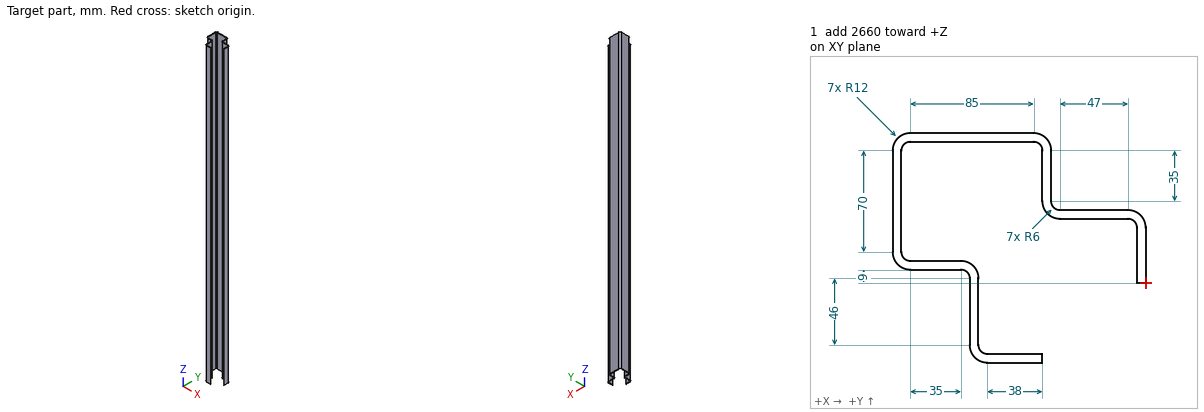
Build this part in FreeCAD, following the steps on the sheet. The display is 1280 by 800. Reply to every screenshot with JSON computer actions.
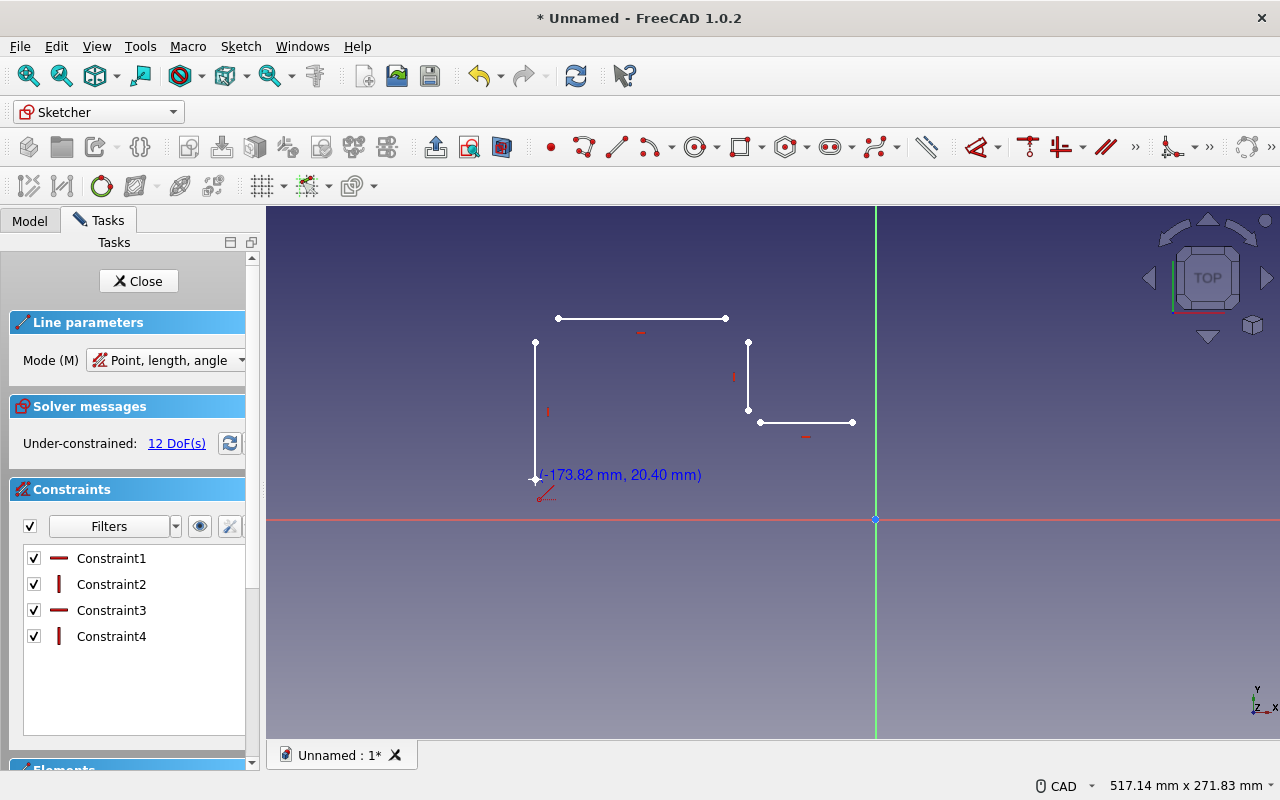
{"action": "left_click", "coordinate": [558, 502]}
{"action": "left_click", "coordinate": [627, 502]}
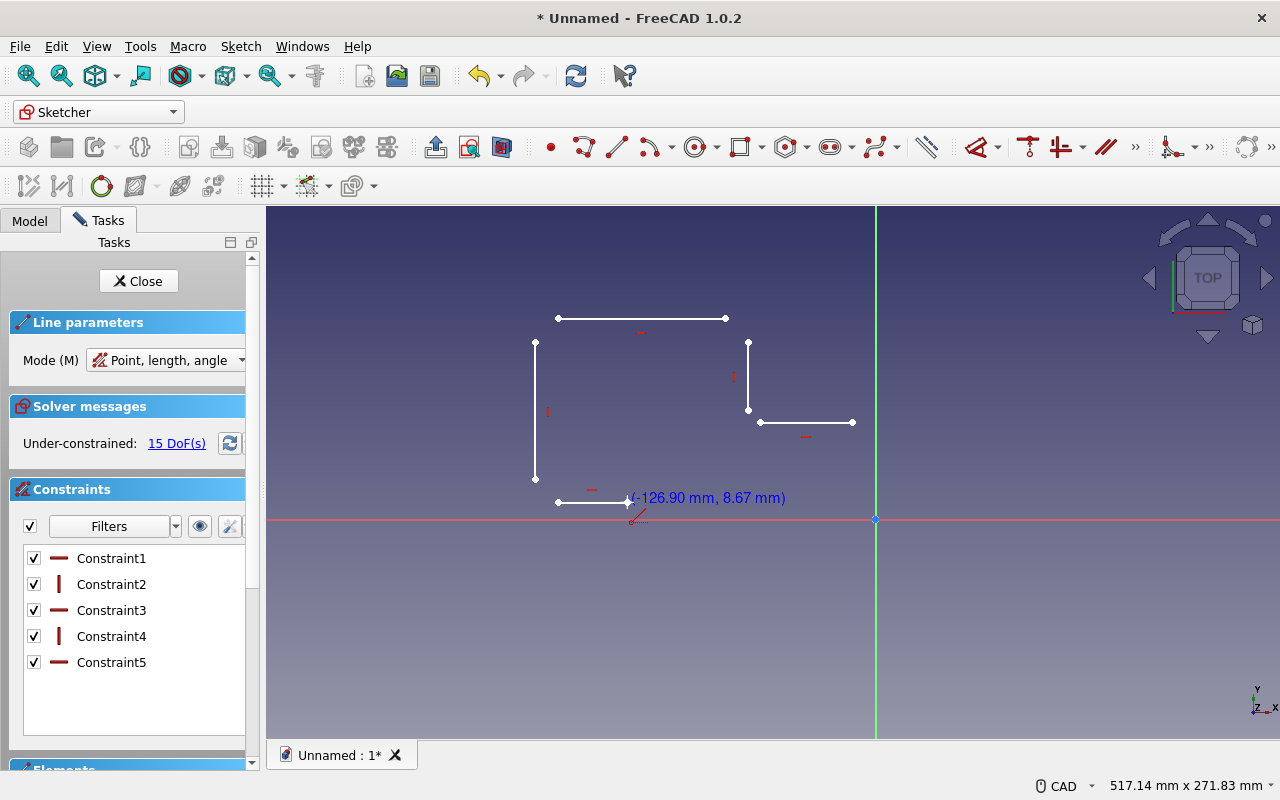
{"action": "scroll", "coordinate": [639, 514], "scroll_direction": "up", "scroll_amount": 5}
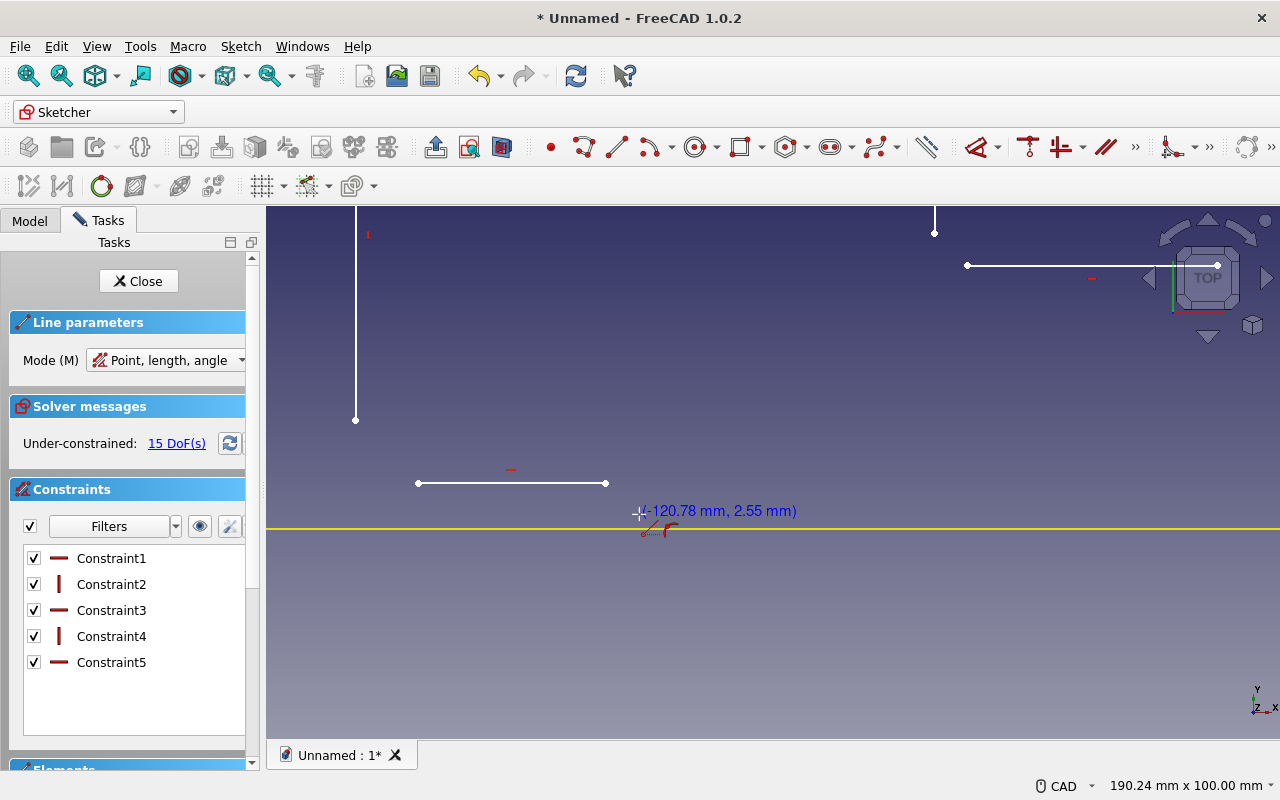
{"action": "left_click", "coordinate": [637, 513]}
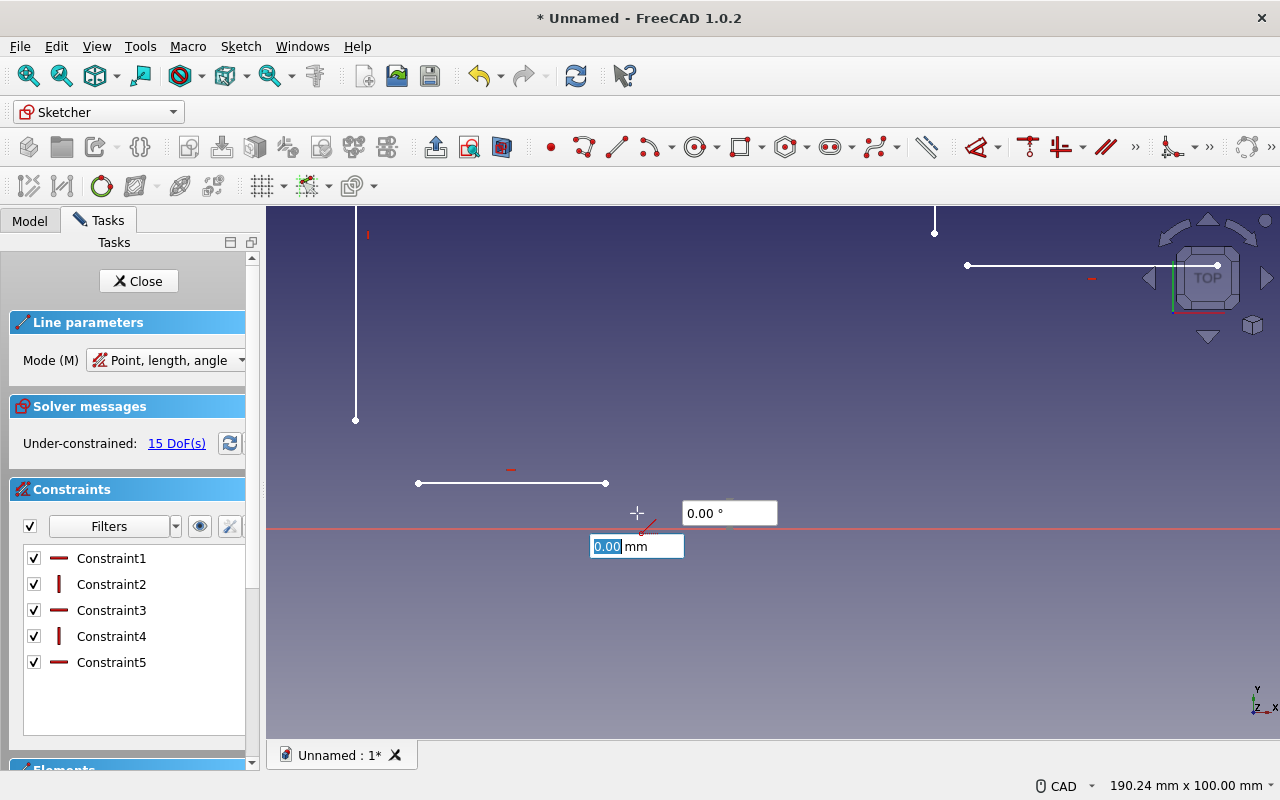
{"action": "scroll", "coordinate": [638, 514], "scroll_direction": "down", "scroll_amount": 5}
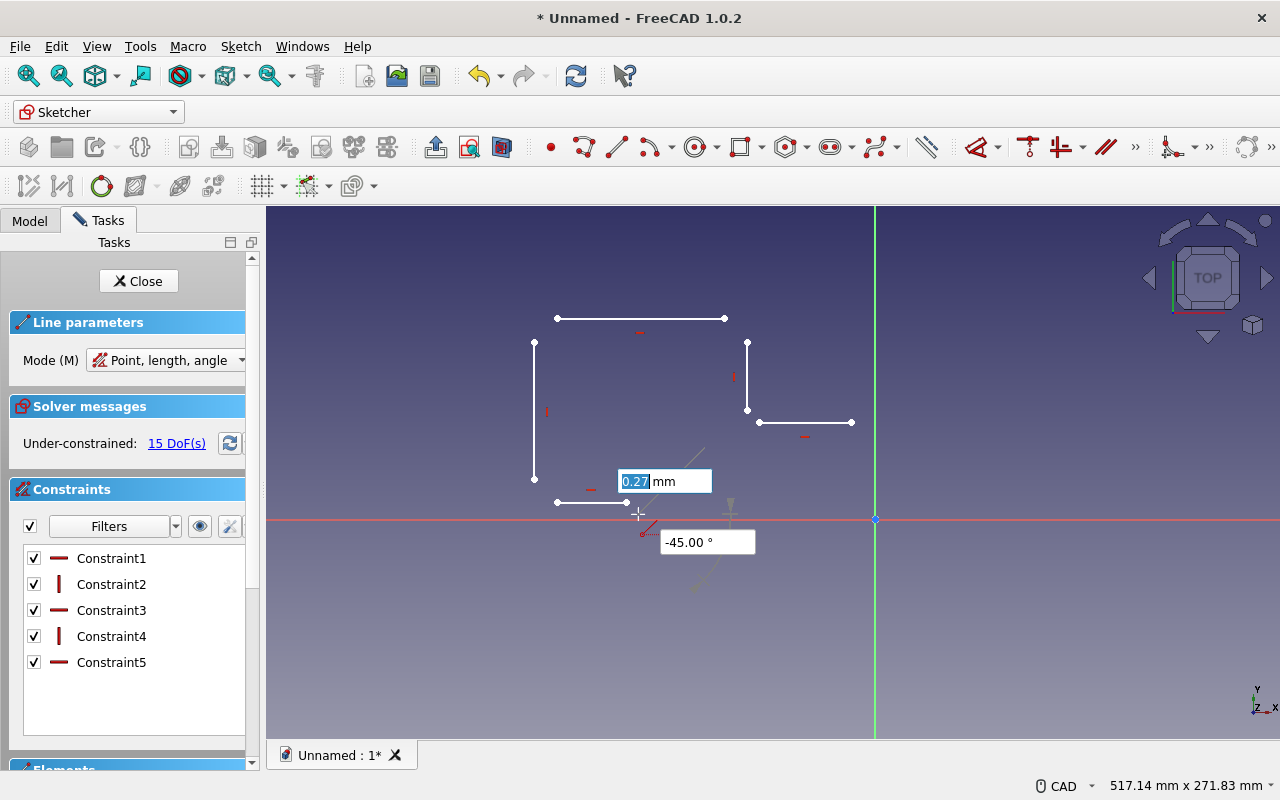
{"action": "left_click", "coordinate": [638, 604]}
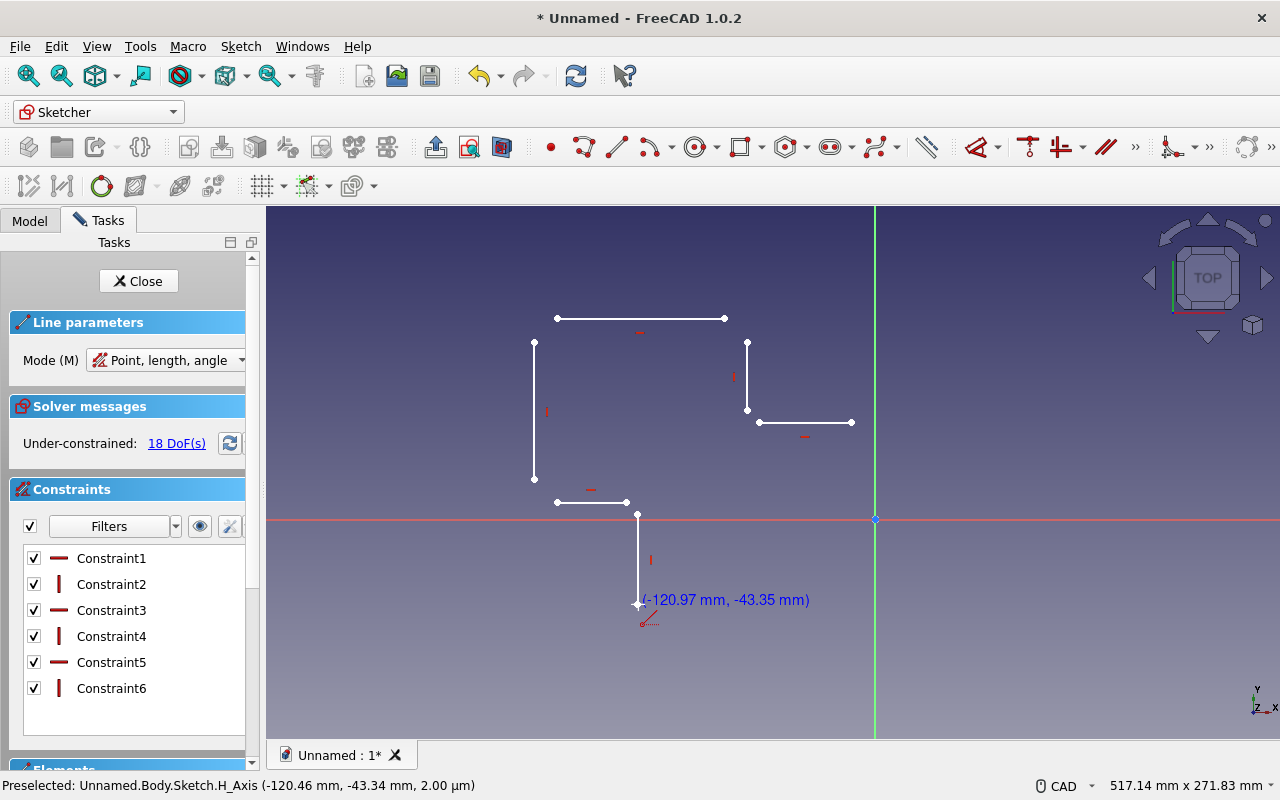
{"action": "key", "text": "g m"}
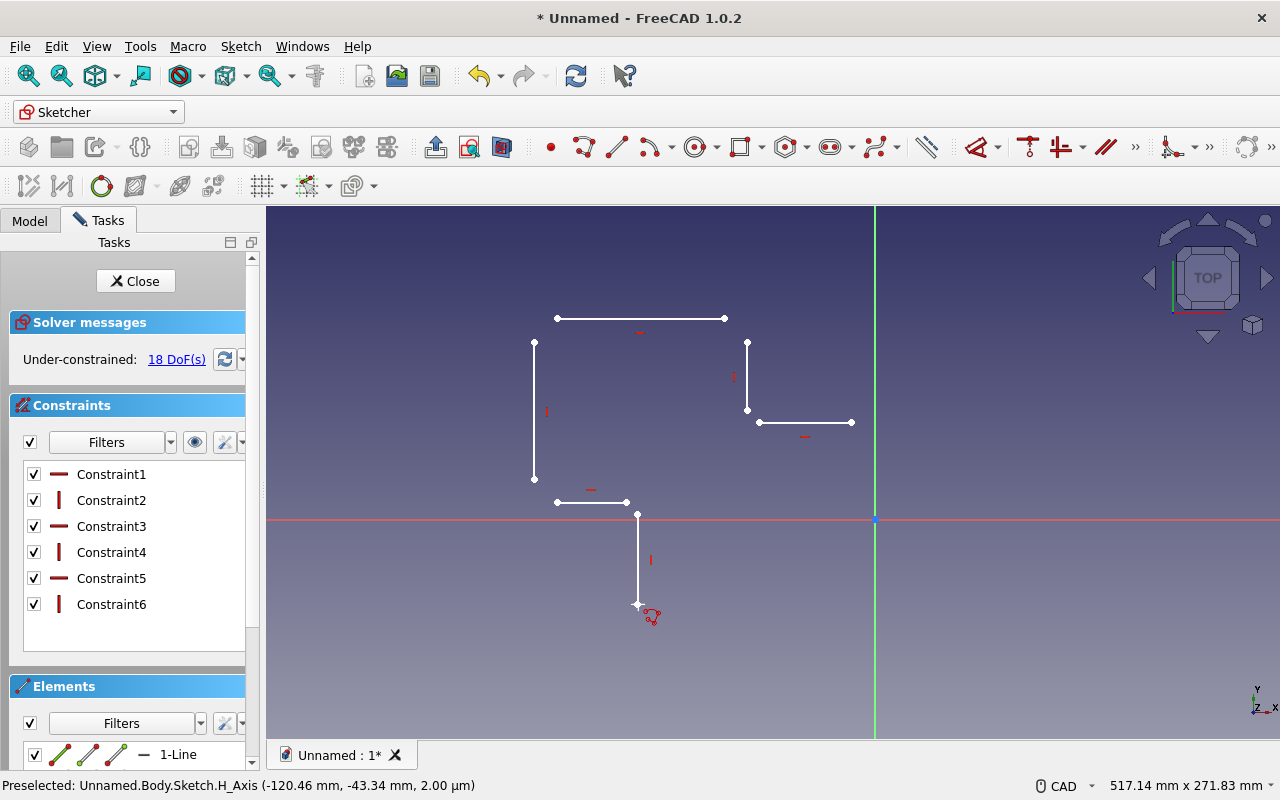
{"action": "left_click", "coordinate": [661, 628]}
{"action": "left_click", "coordinate": [736, 628]}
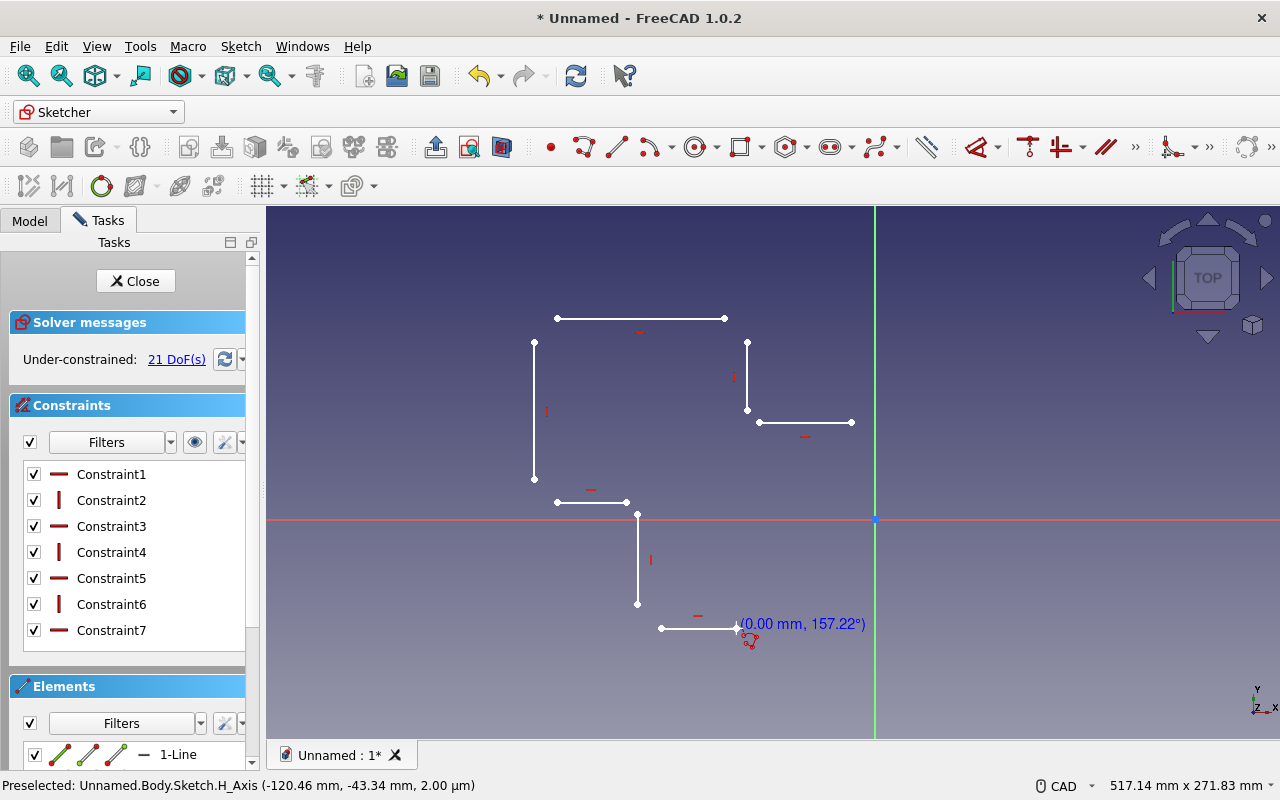
{"action": "scroll", "coordinate": [736, 616], "scroll_direction": "up", "scroll_amount": 2}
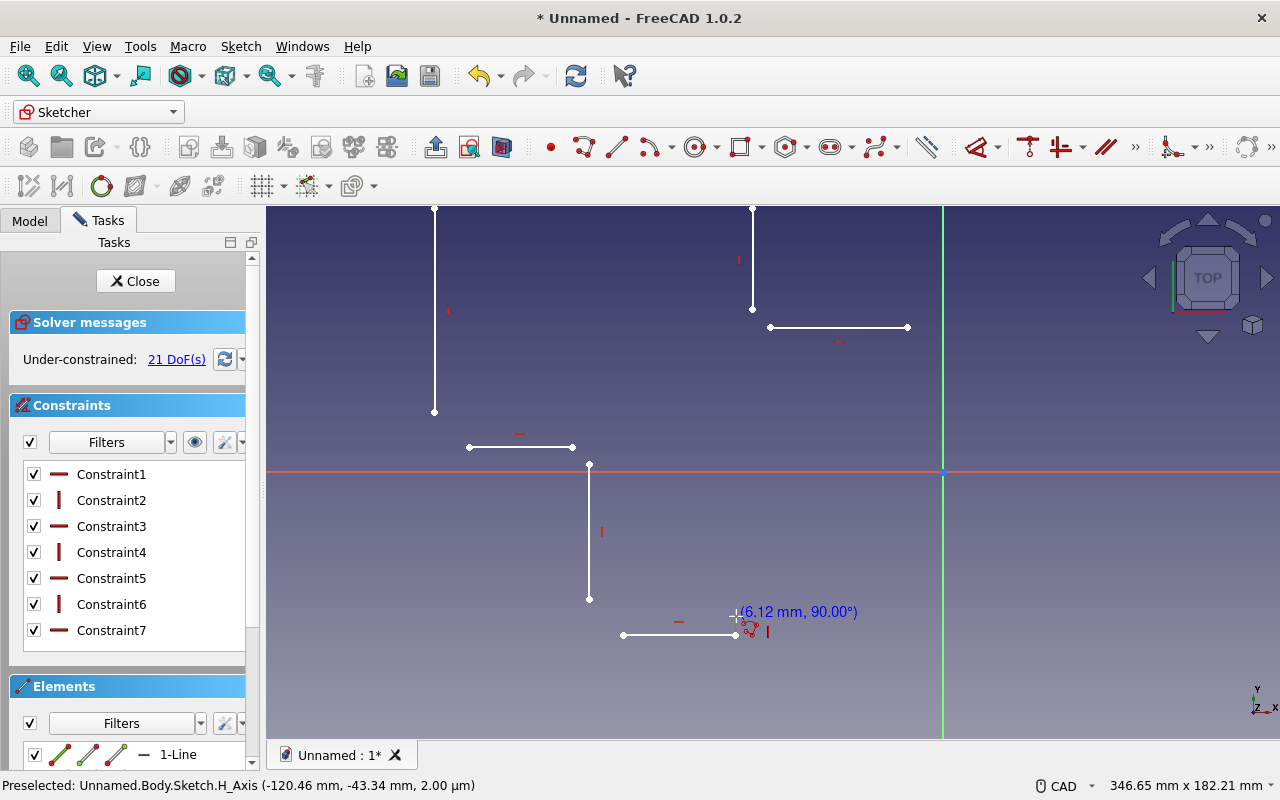
{"action": "left_click", "coordinate": [736, 616]}
{"action": "left_click", "coordinate": [625, 616]}
{"action": "right_click", "coordinate": [625, 616]}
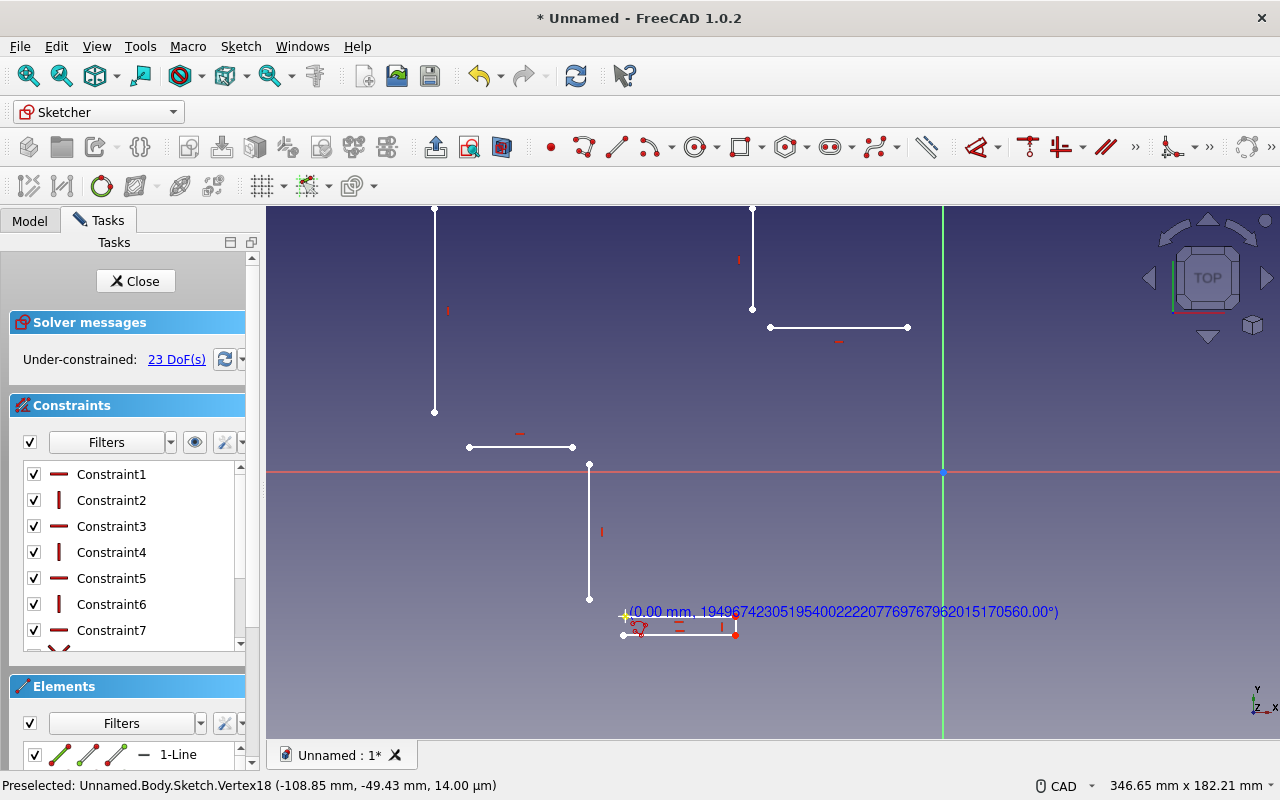
{"action": "key", "text": "g l"}